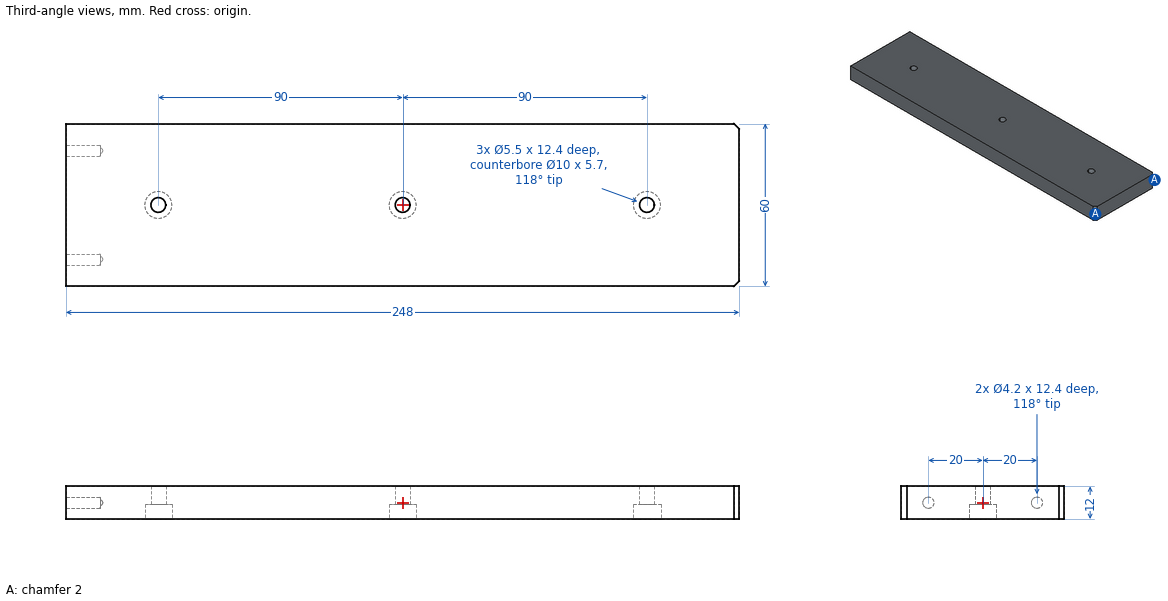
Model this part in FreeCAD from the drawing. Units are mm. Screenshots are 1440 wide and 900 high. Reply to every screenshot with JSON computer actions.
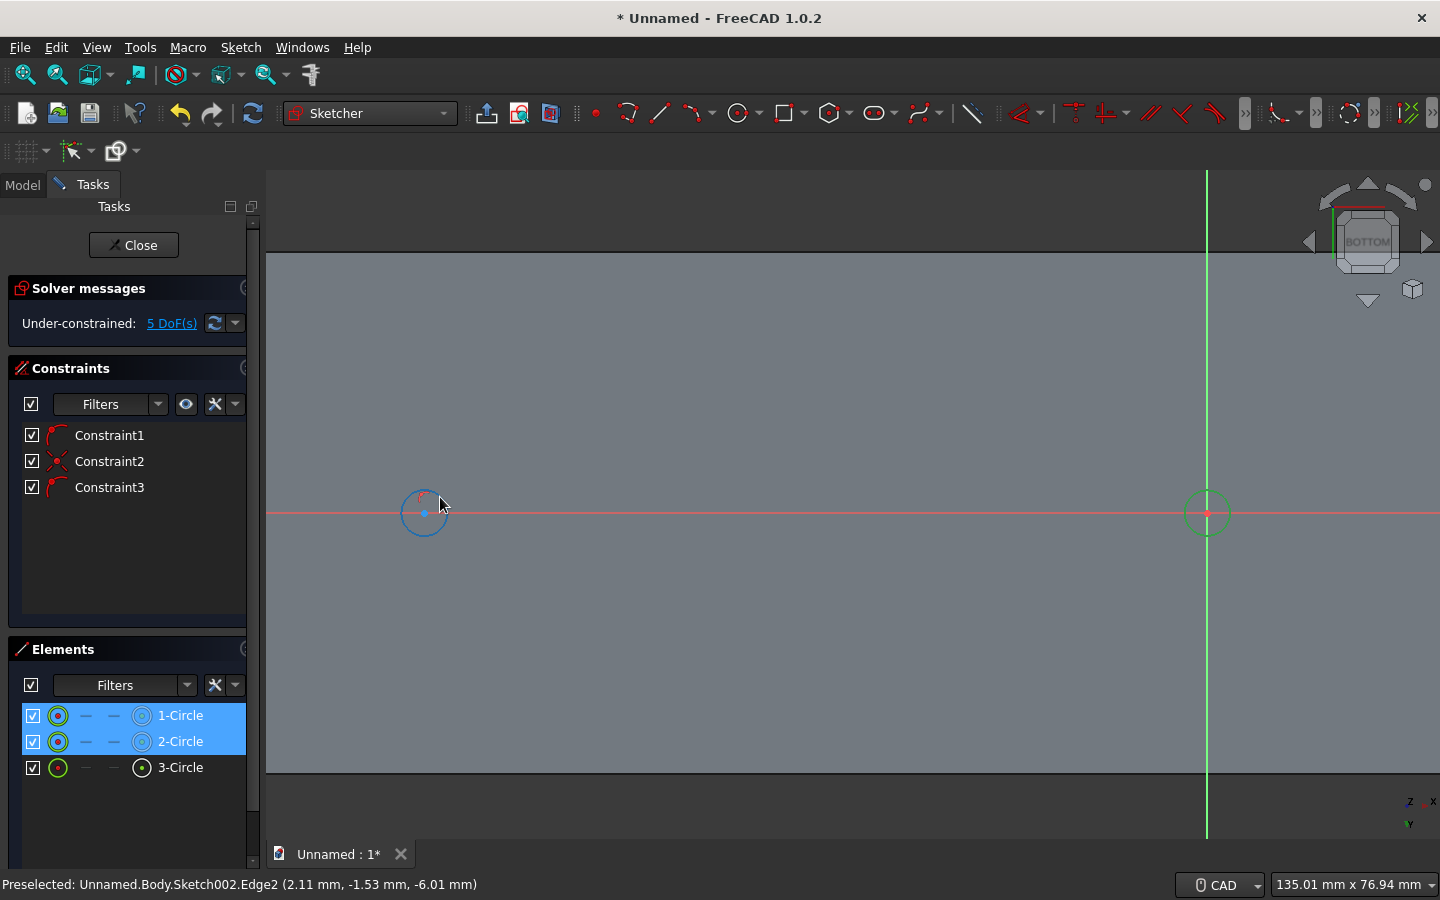
{"action": "left_click", "coordinate": [441, 497]}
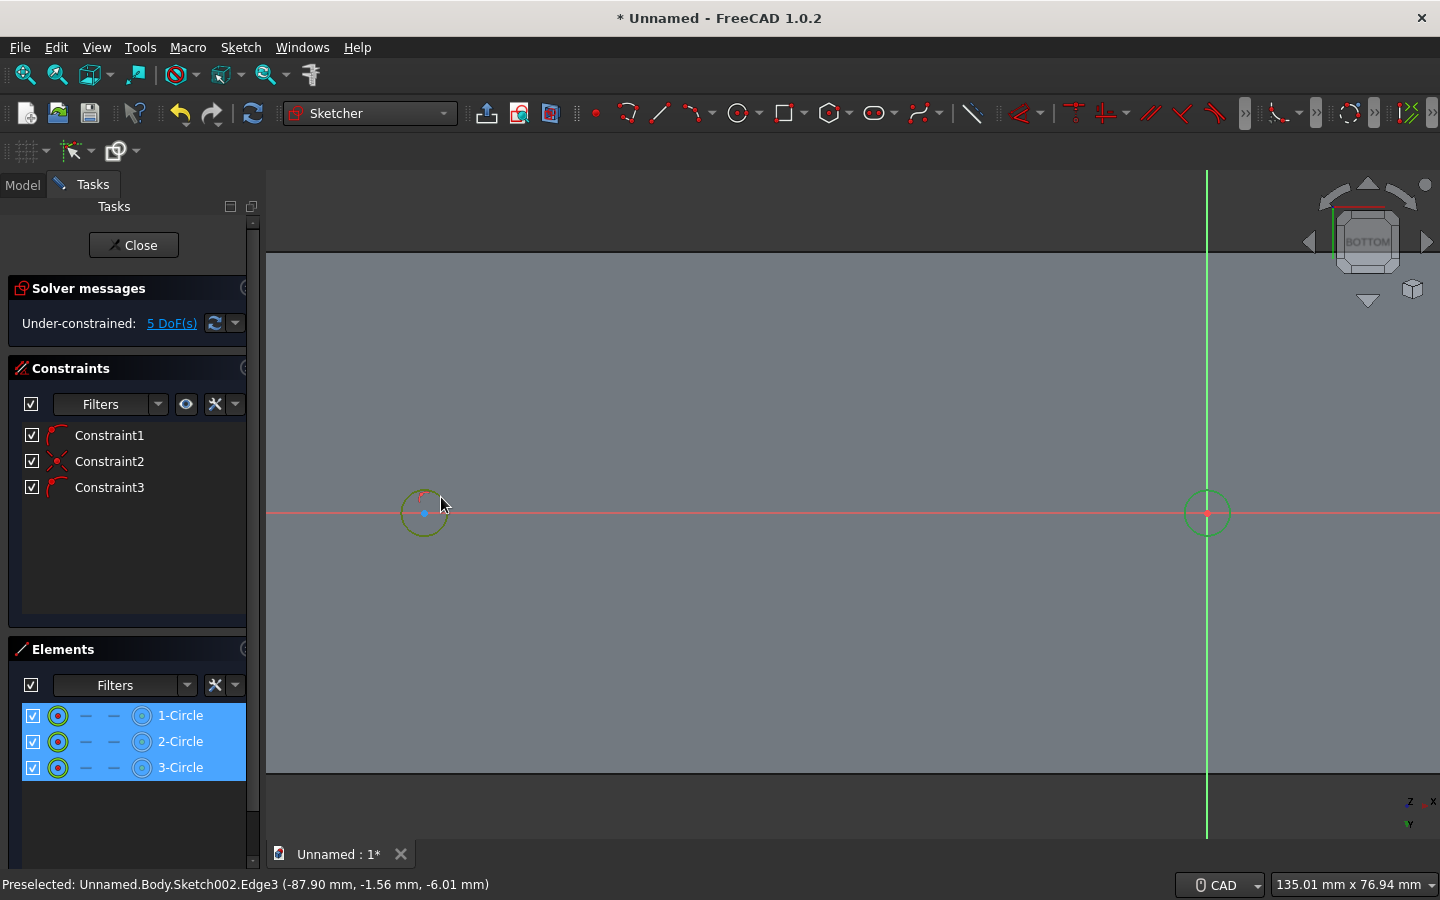
{"action": "key", "text": "e"}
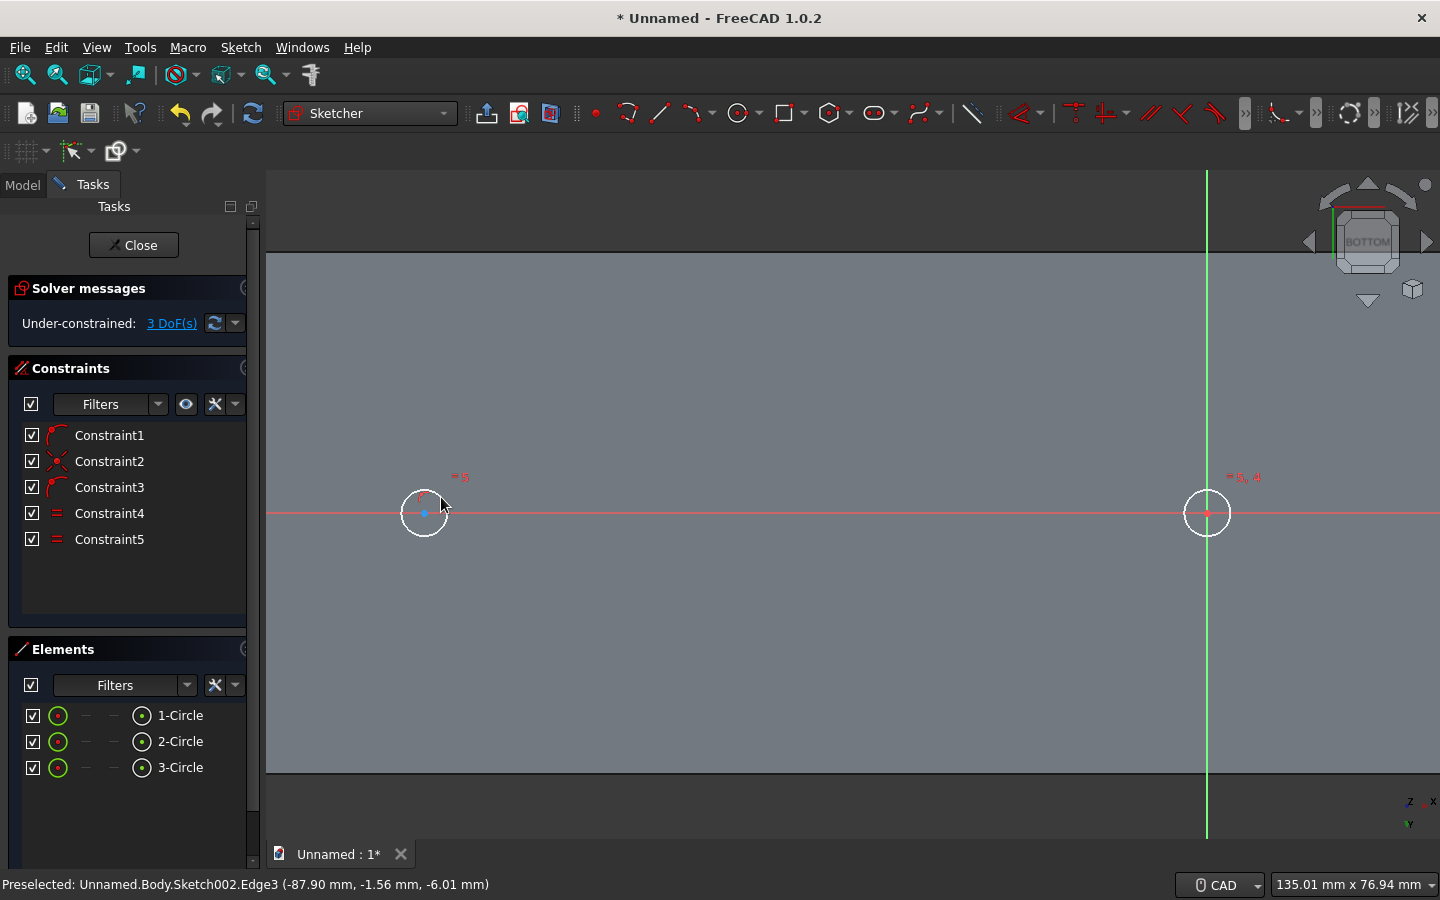
{"action": "left_click", "coordinate": [1020, 114]}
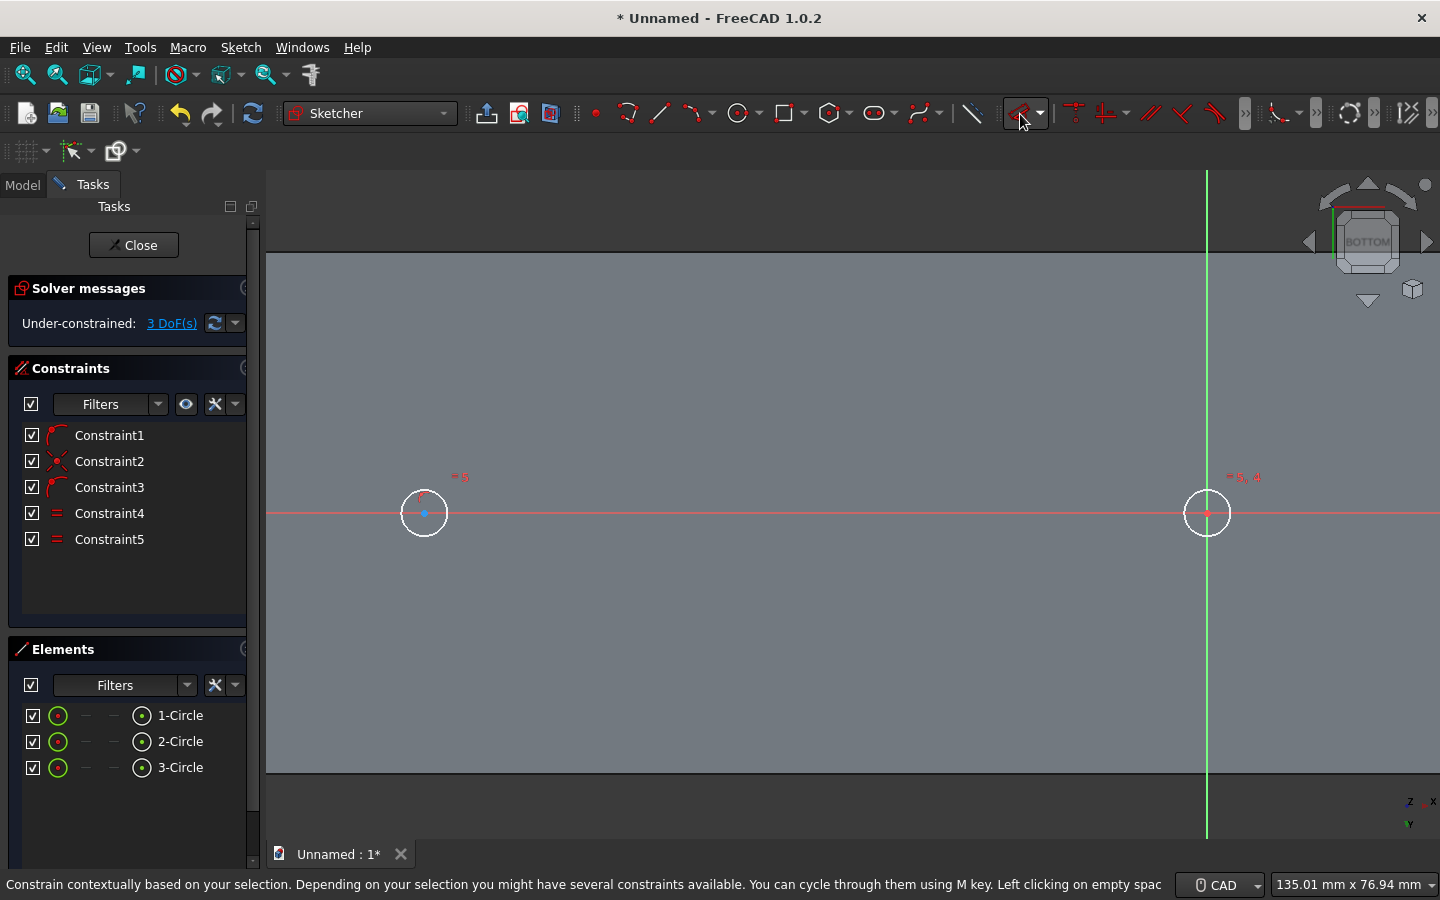
{"action": "scroll", "coordinate": [439, 497], "scroll_direction": "down", "scroll_amount": 4}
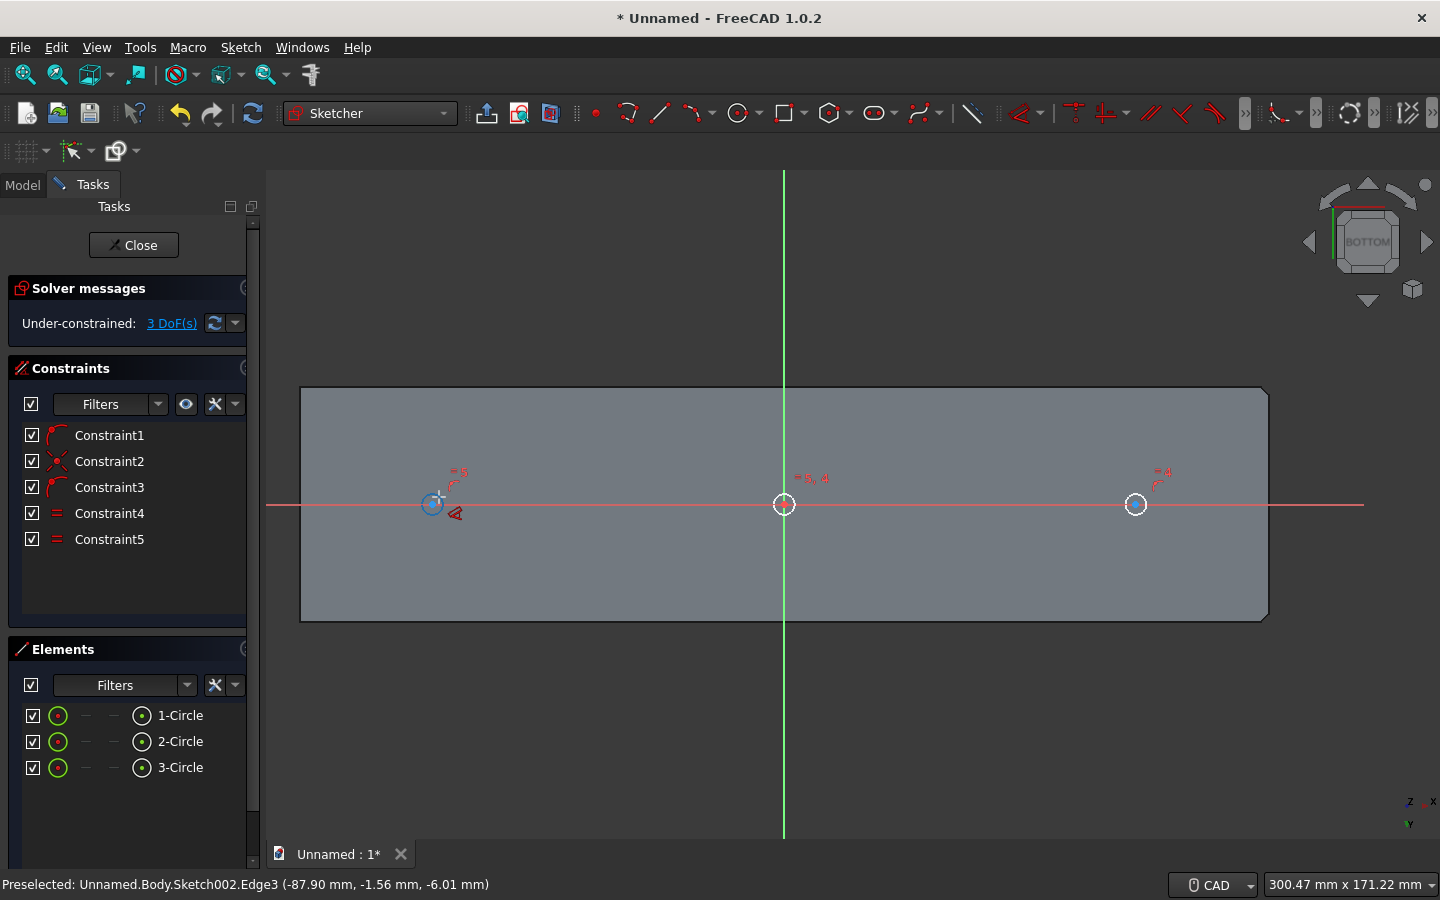
{"action": "scroll", "coordinate": [1143, 497], "scroll_direction": "up", "scroll_amount": 4}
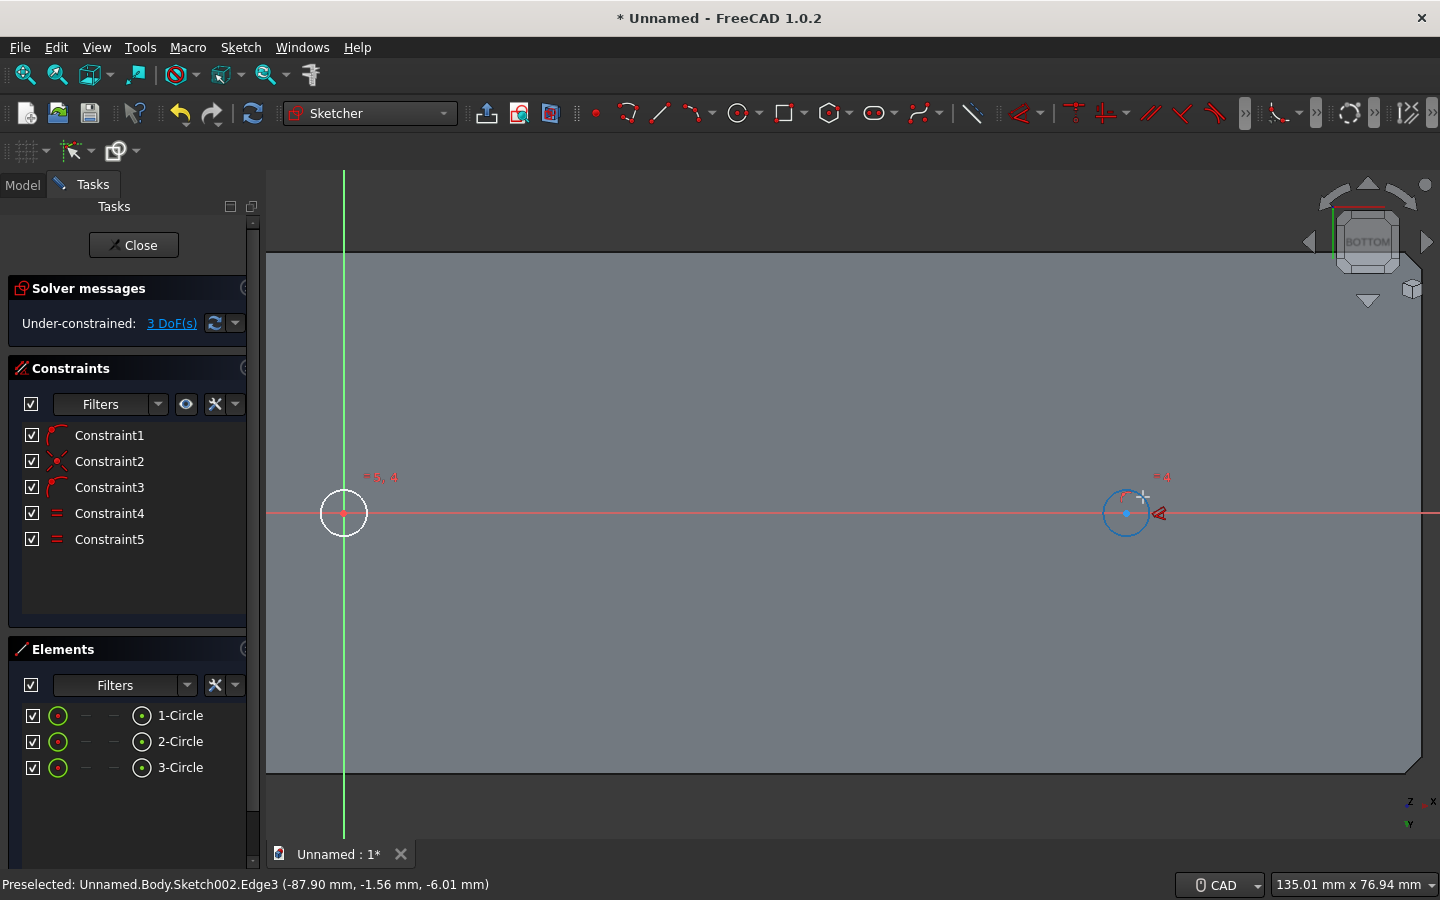
{"action": "left_click", "coordinate": [1143, 497]}
{"action": "left_click", "coordinate": [1166, 475]}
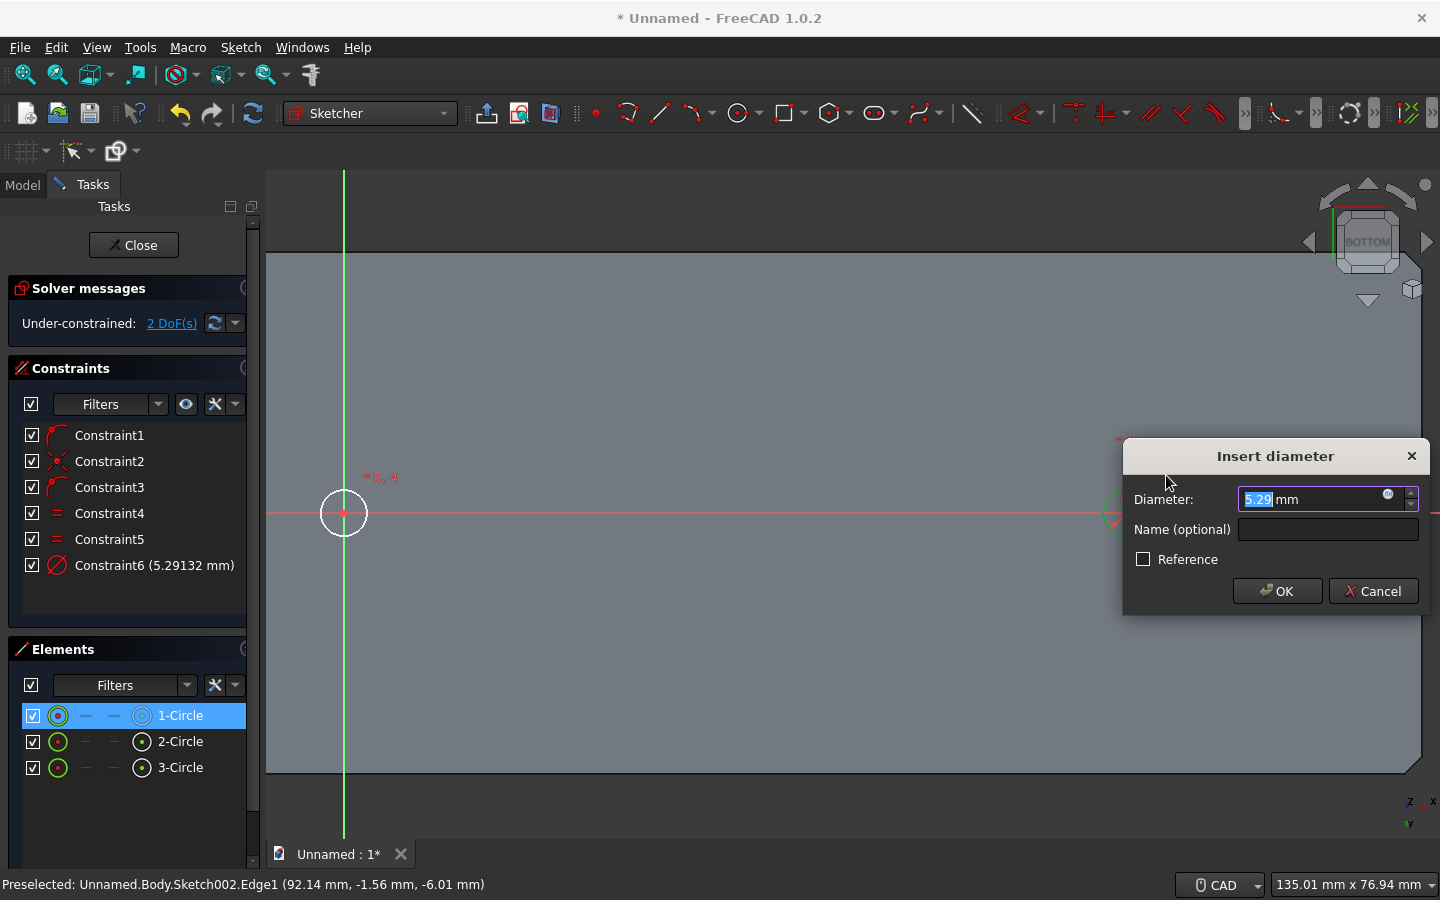
{"action": "type", "text": "5.5"}
{"action": "key", "text": "Return"}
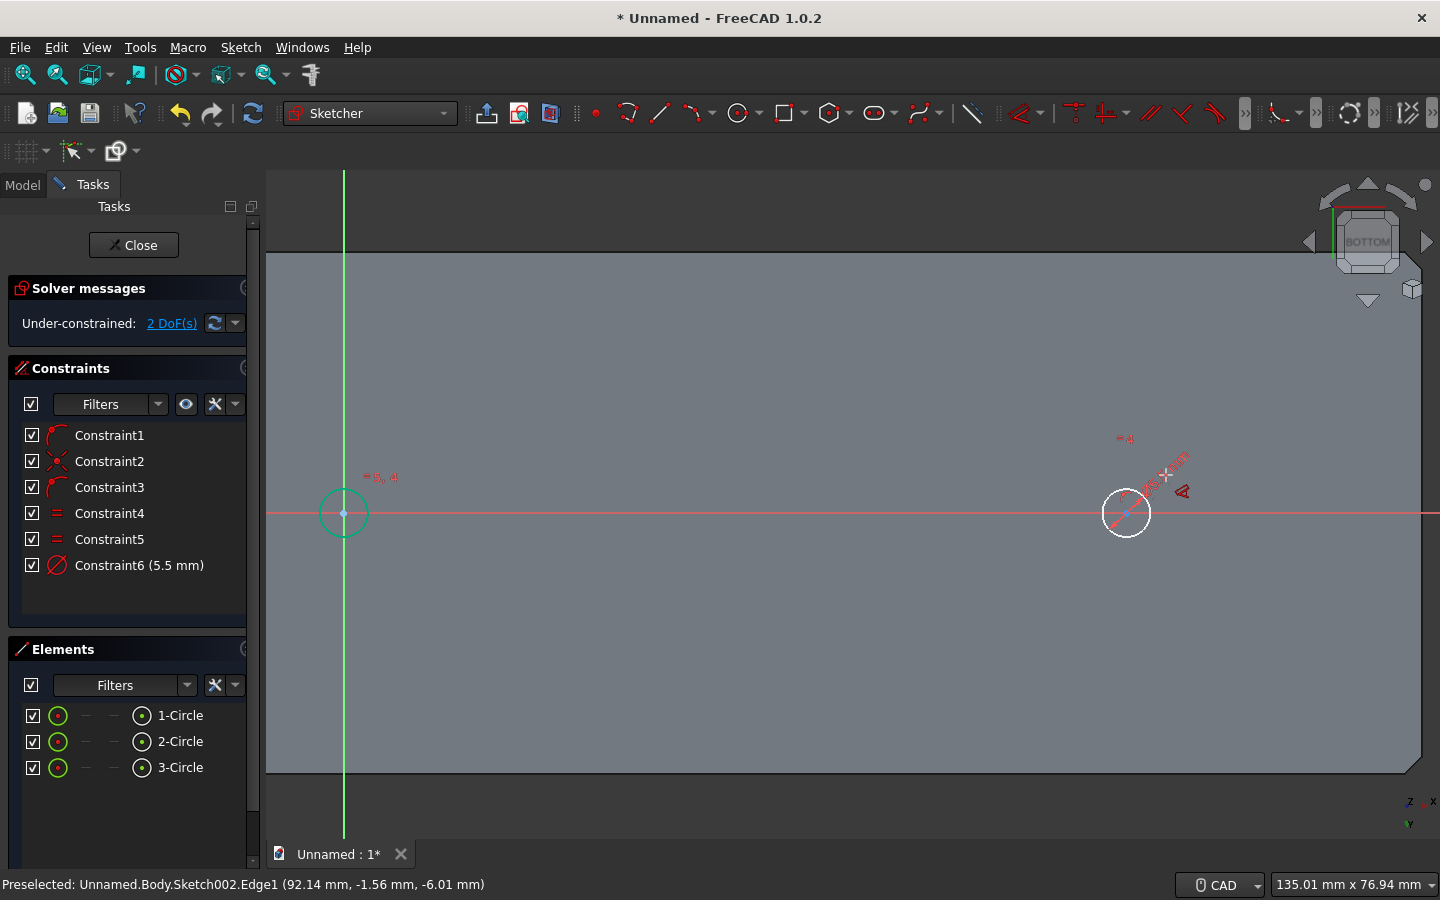
{"action": "left_click", "coordinate": [1126, 513]}
{"action": "left_click", "coordinate": [735, 547]}